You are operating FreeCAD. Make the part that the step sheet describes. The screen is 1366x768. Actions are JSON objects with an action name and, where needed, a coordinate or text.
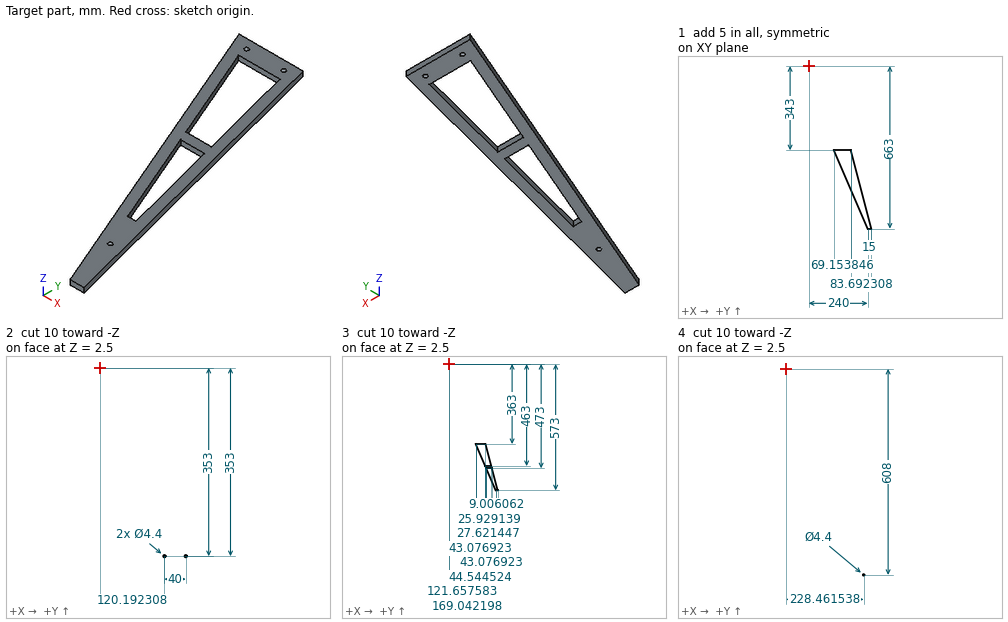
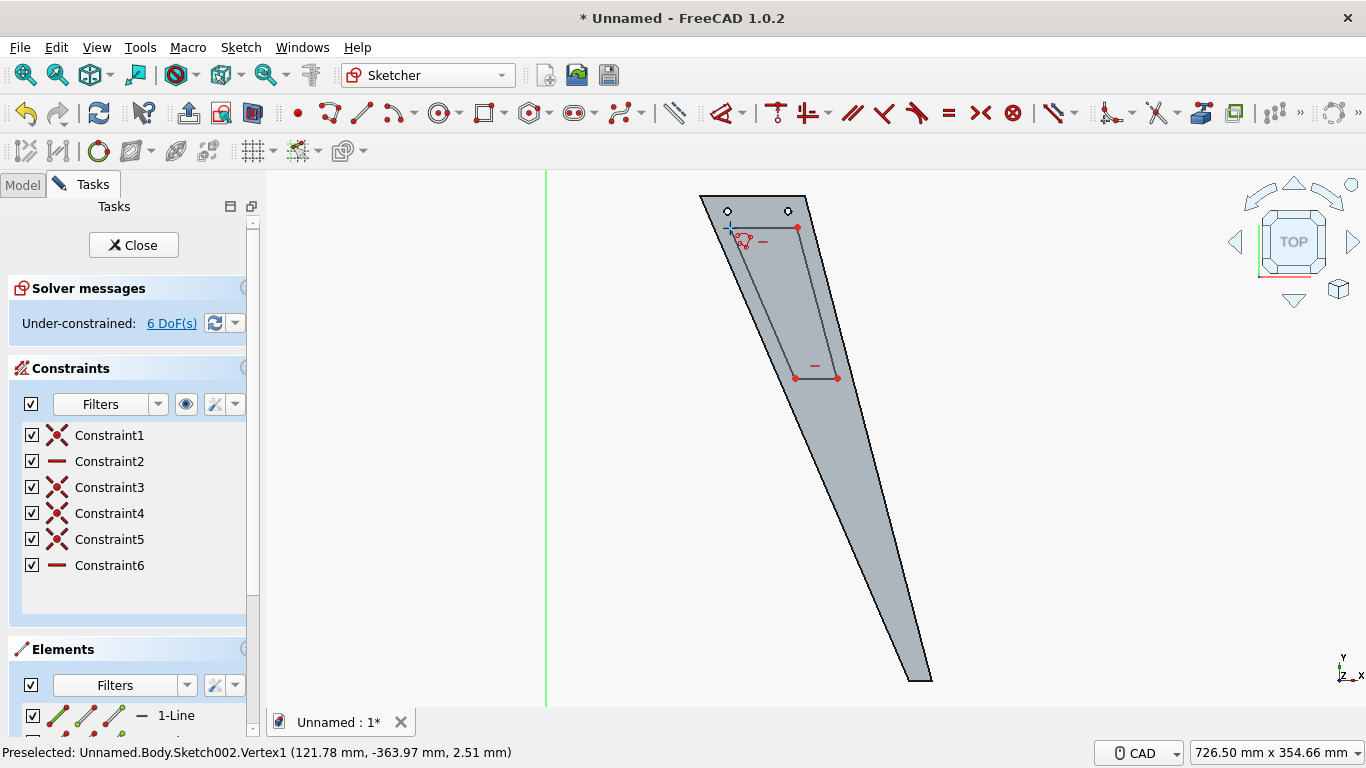
{"action": "left_click", "coordinate": [802, 393]}
{"action": "left_click", "coordinate": [867, 544]}
{"action": "left_click", "coordinate": [880, 544]}
{"action": "left_click", "coordinate": [841, 393]}
{"action": "left_click", "coordinate": [802, 394]}
{"action": "key", "text": "Escape"}
{"action": "key", "text": "Escape"}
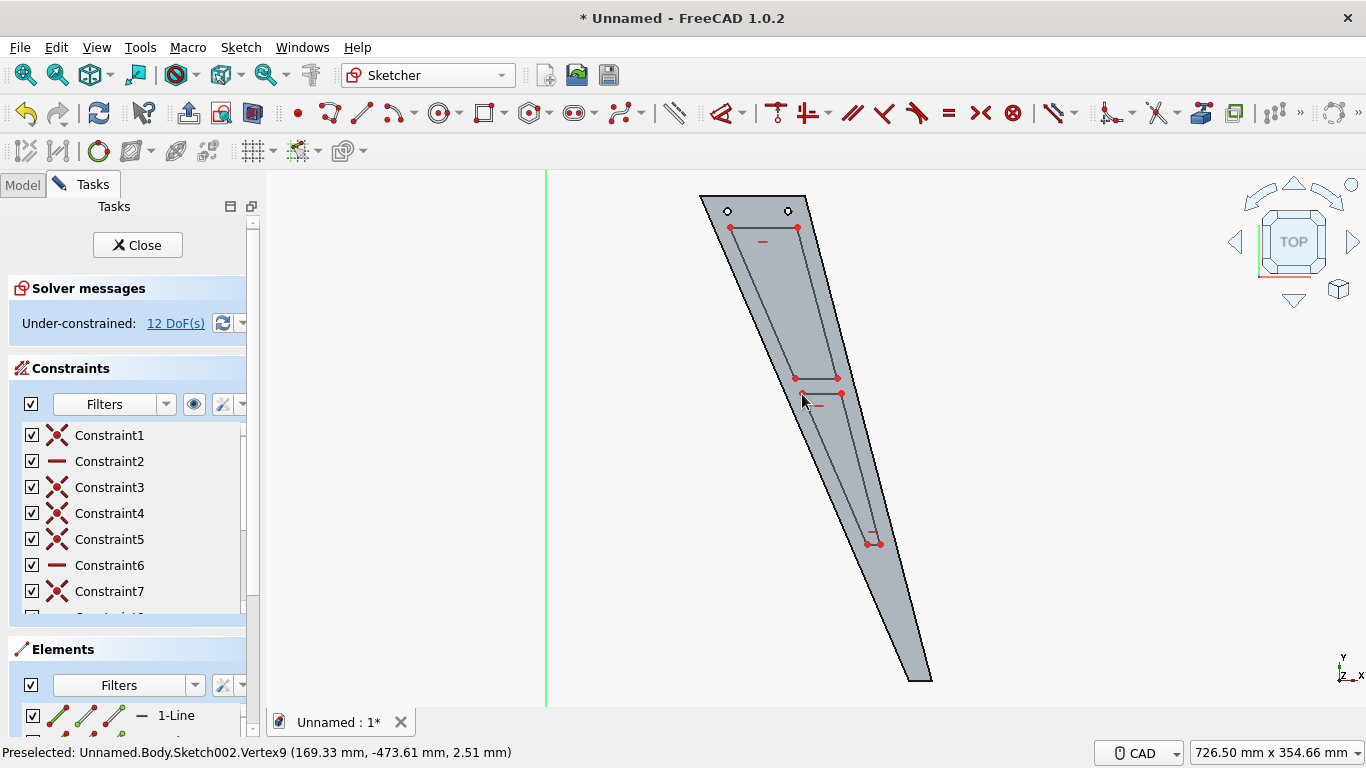
{"action": "left_click", "coordinate": [722, 114]}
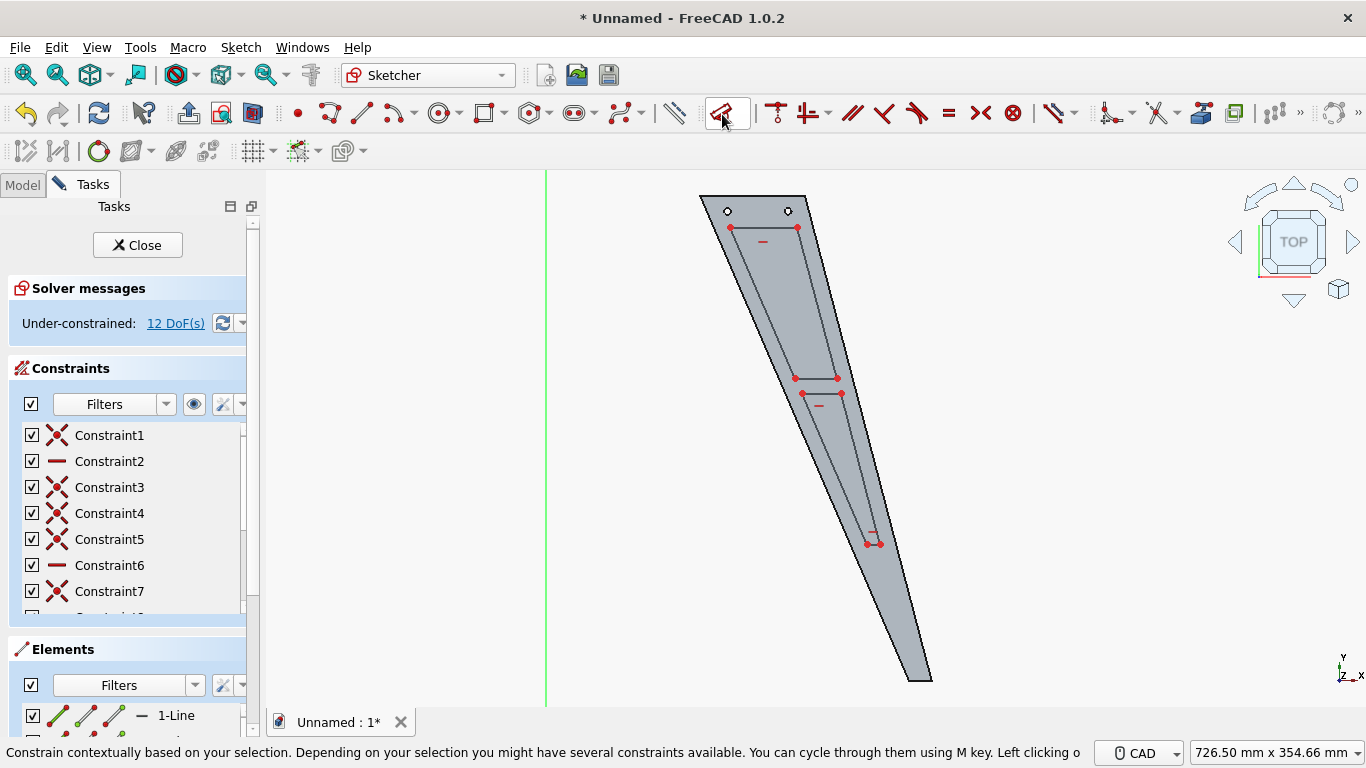
{"action": "left_click", "coordinate": [730, 228]}
{"action": "left_click", "coordinate": [512, 213]}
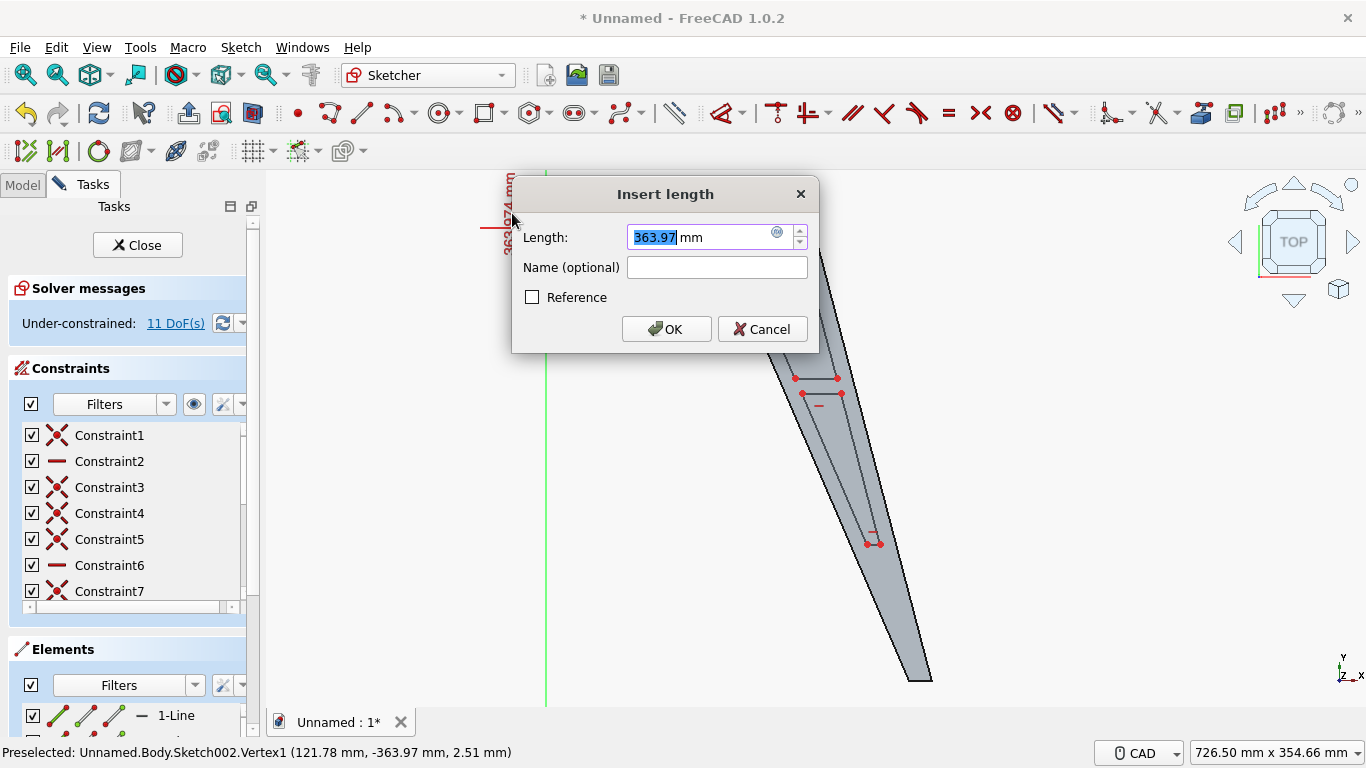
{"action": "type", "text": "363"}
{"action": "key", "text": "Return"}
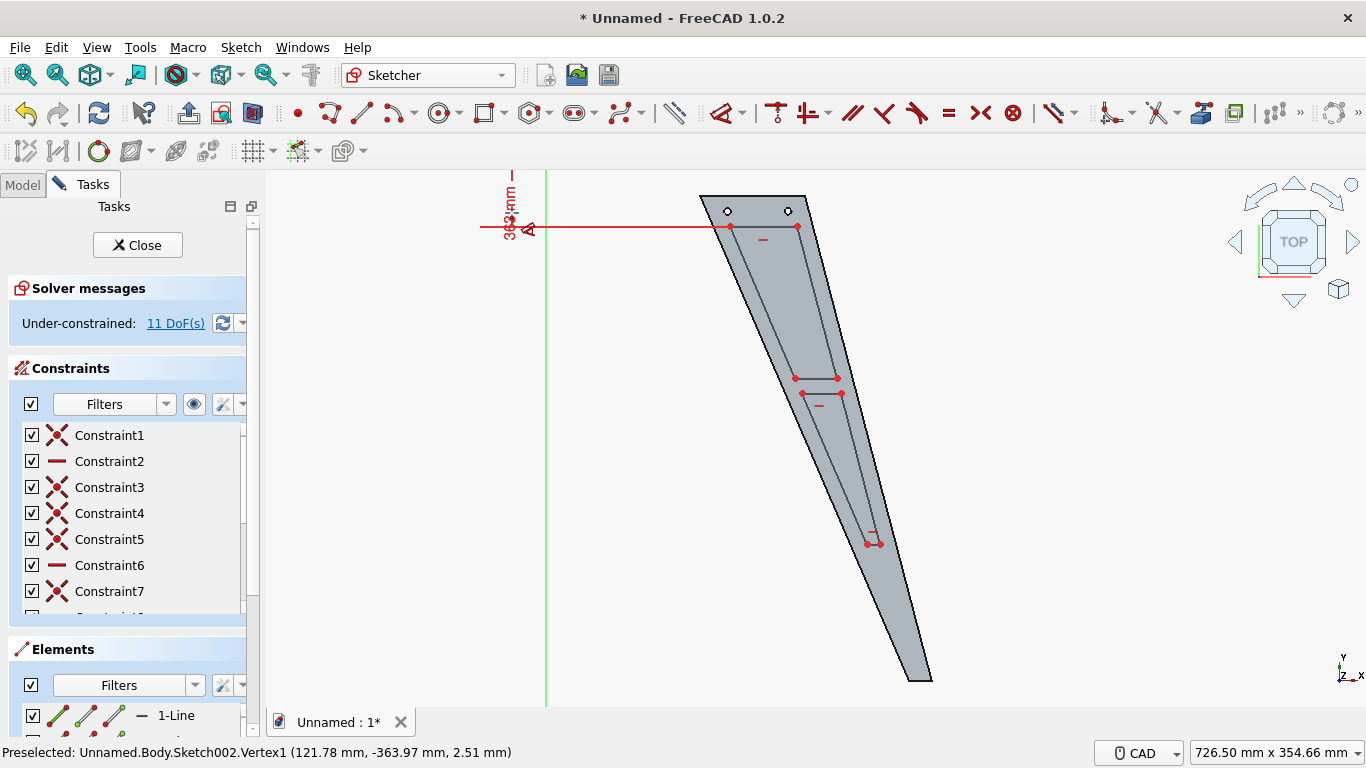
{"action": "left_click", "coordinate": [795, 379]}
{"action": "left_click", "coordinate": [512, 289]}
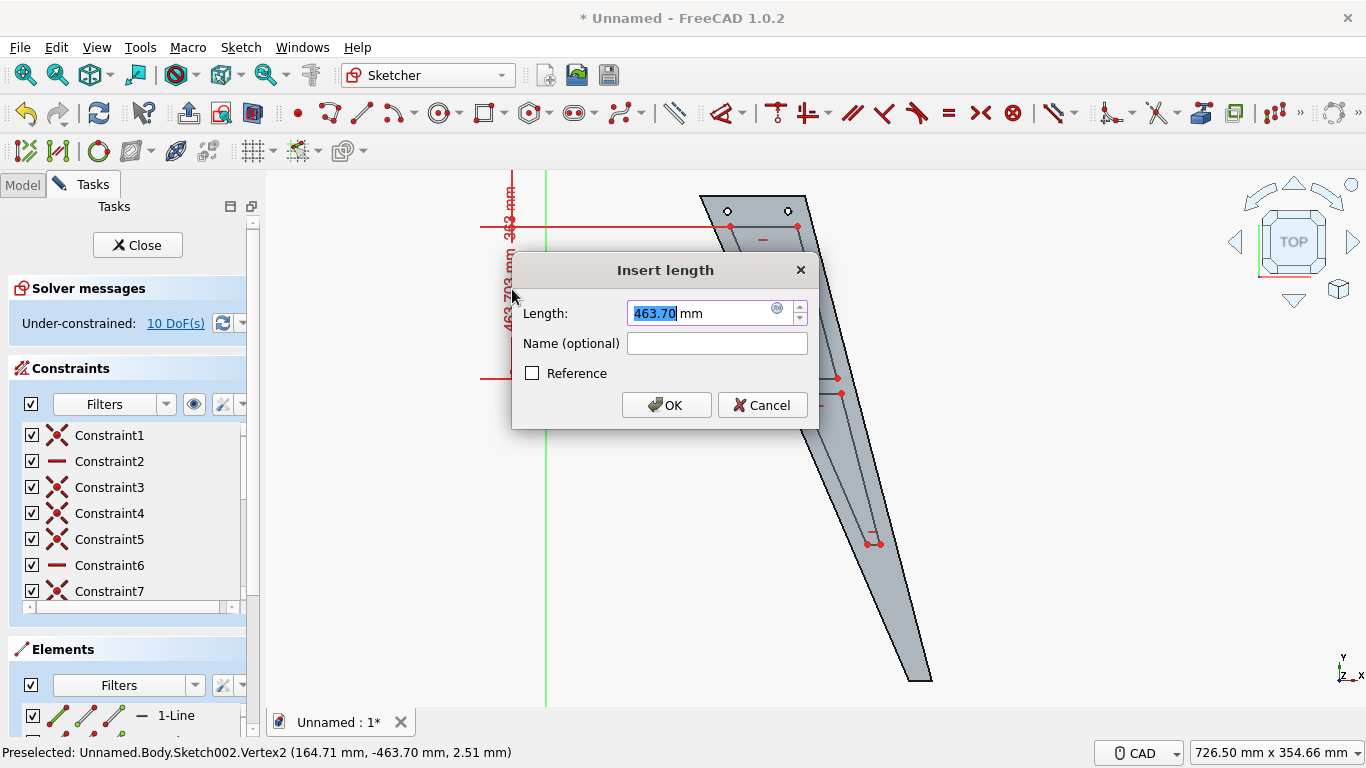
{"action": "type", "text": "463"}
{"action": "key", "text": "Return"}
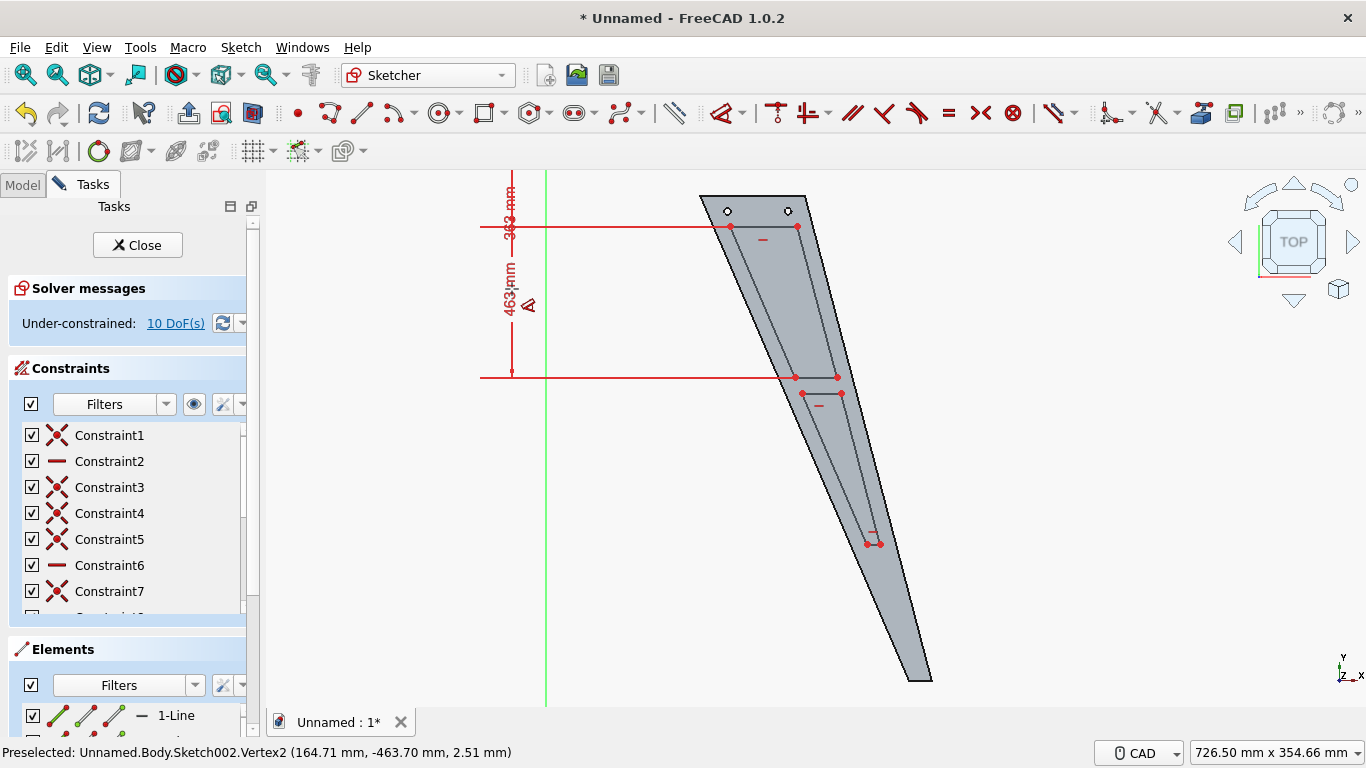
{"action": "left_click", "coordinate": [802, 394]}
{"action": "left_click", "coordinate": [512, 251]}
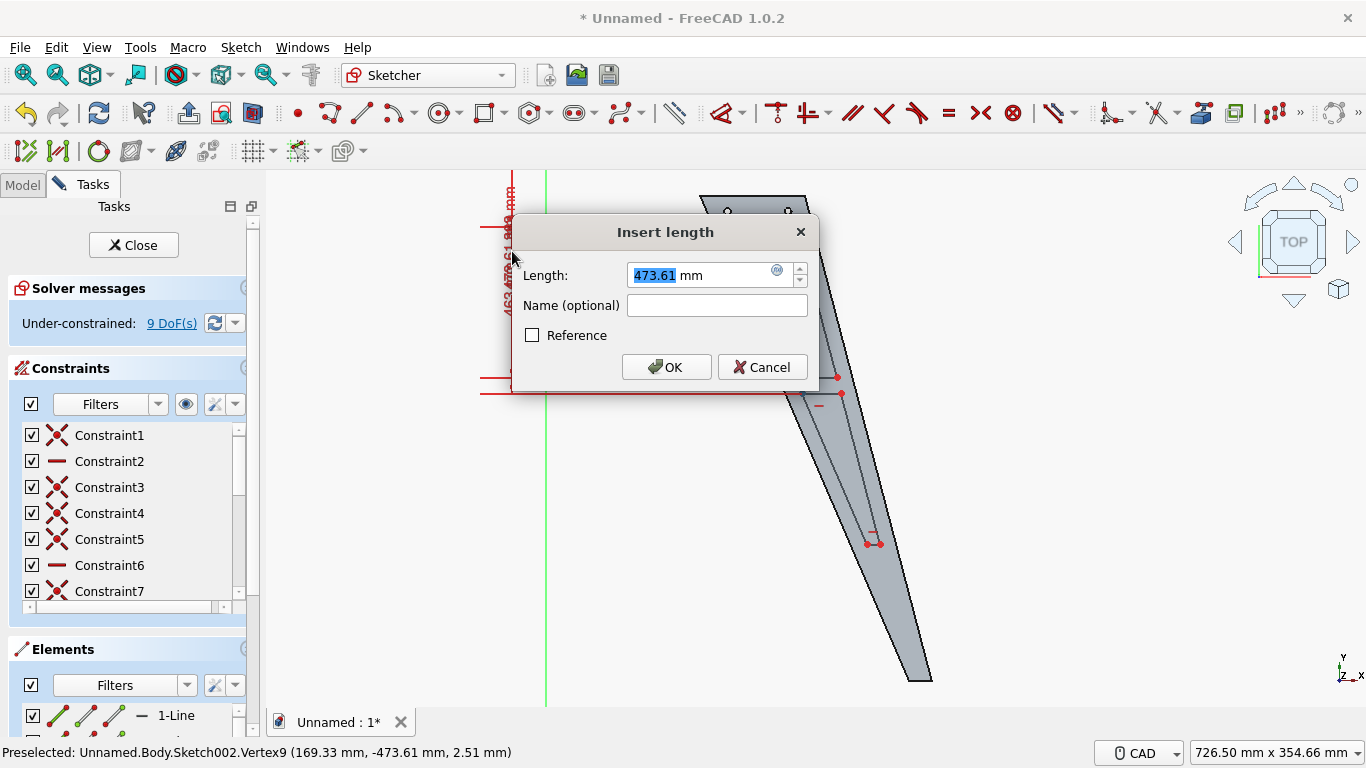
{"action": "type", "text": "473"}
{"action": "key", "text": "Return"}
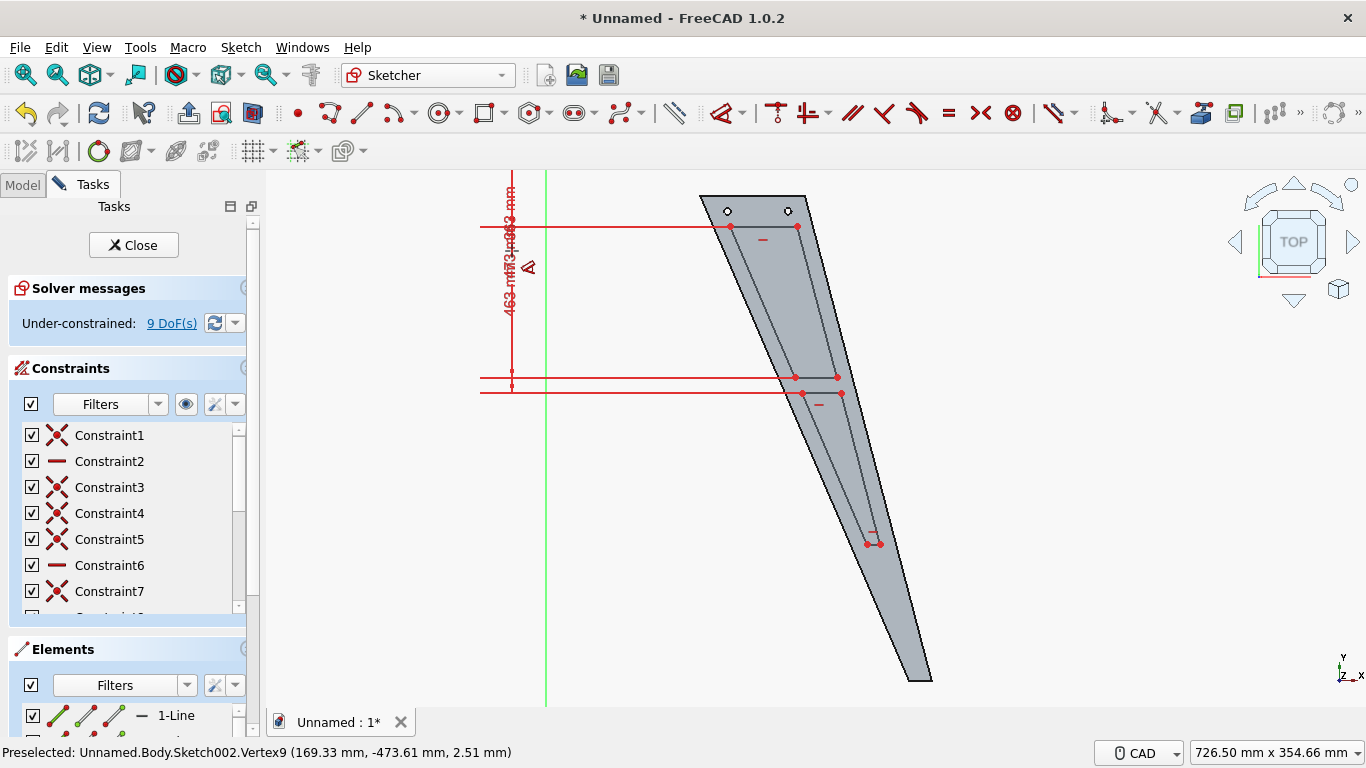
{"action": "left_click", "coordinate": [867, 545]}
{"action": "left_click", "coordinate": [512, 372]}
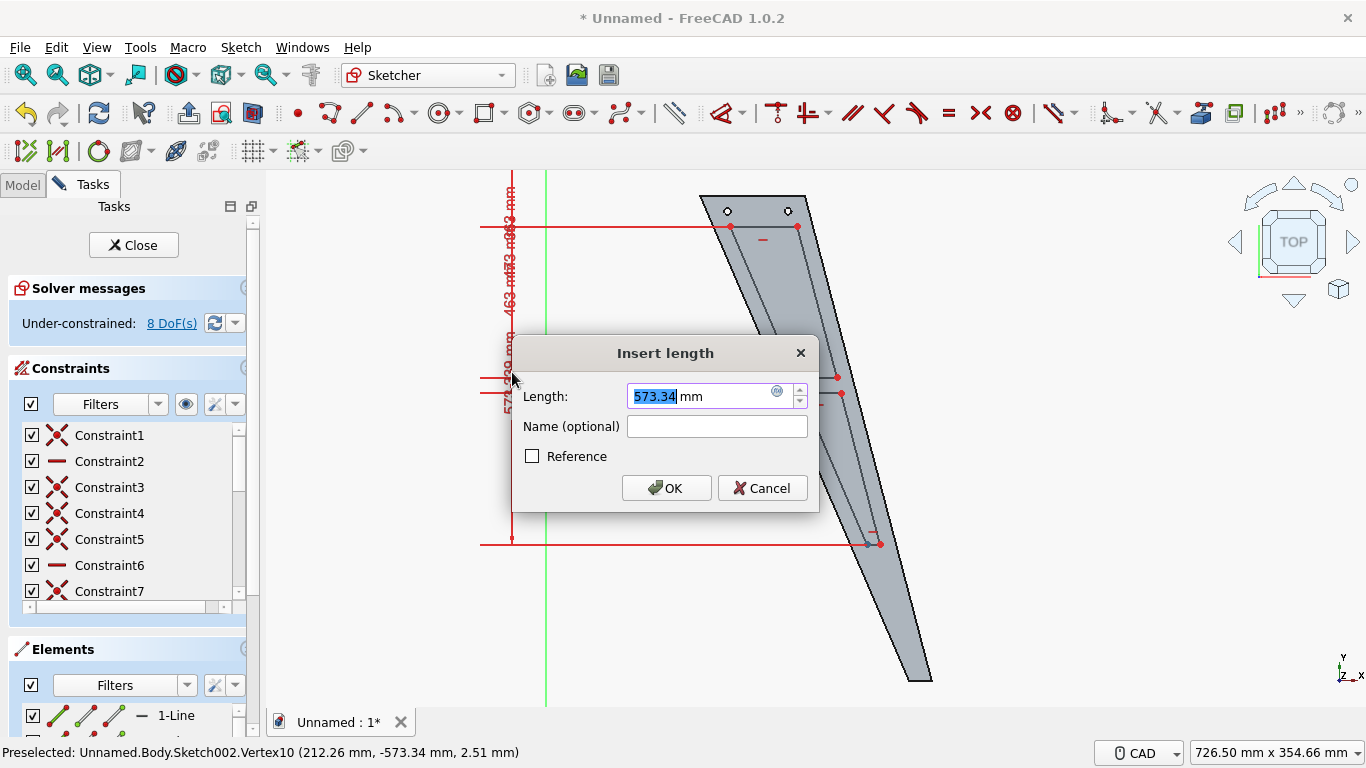
{"action": "type", "text": "573"}
{"action": "key", "text": "Return"}